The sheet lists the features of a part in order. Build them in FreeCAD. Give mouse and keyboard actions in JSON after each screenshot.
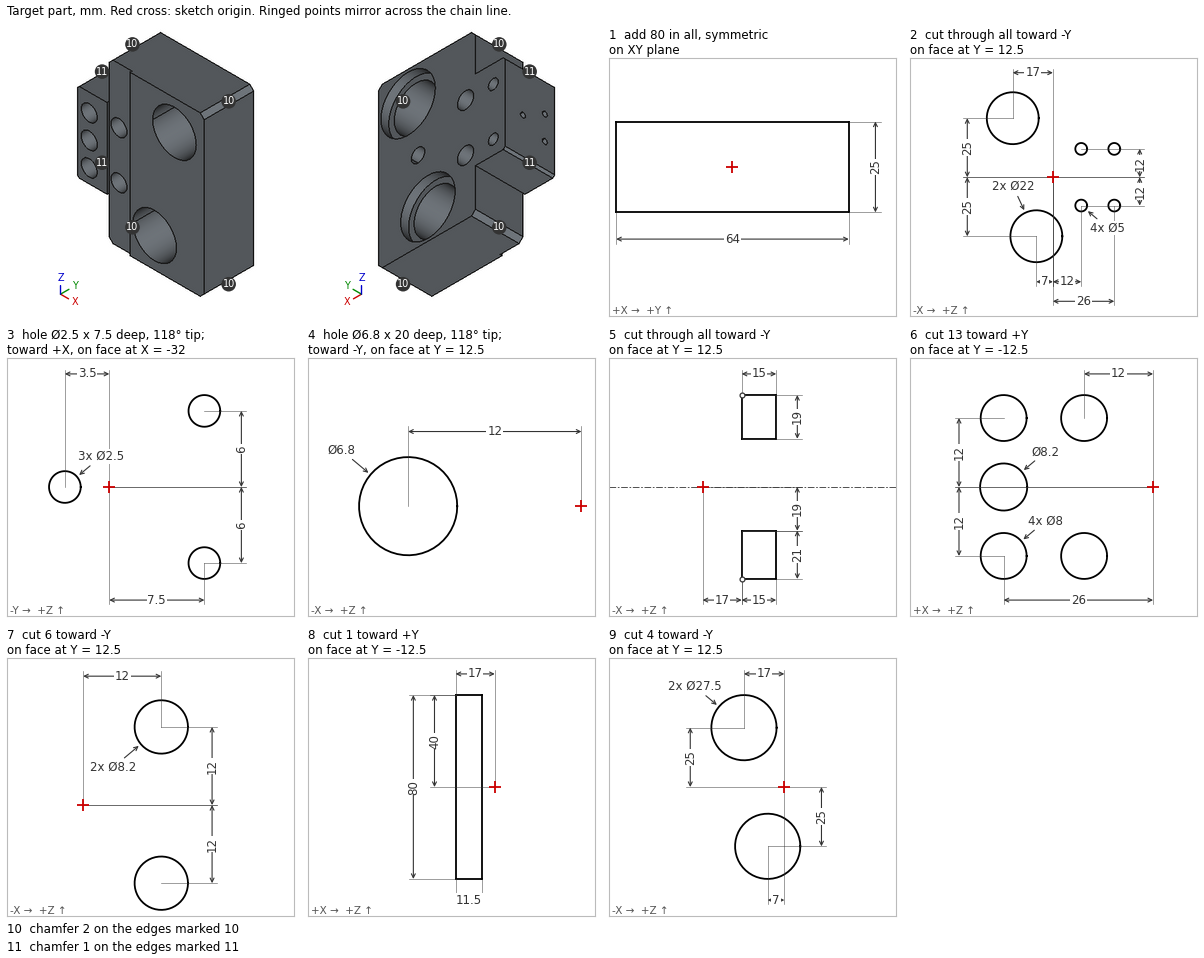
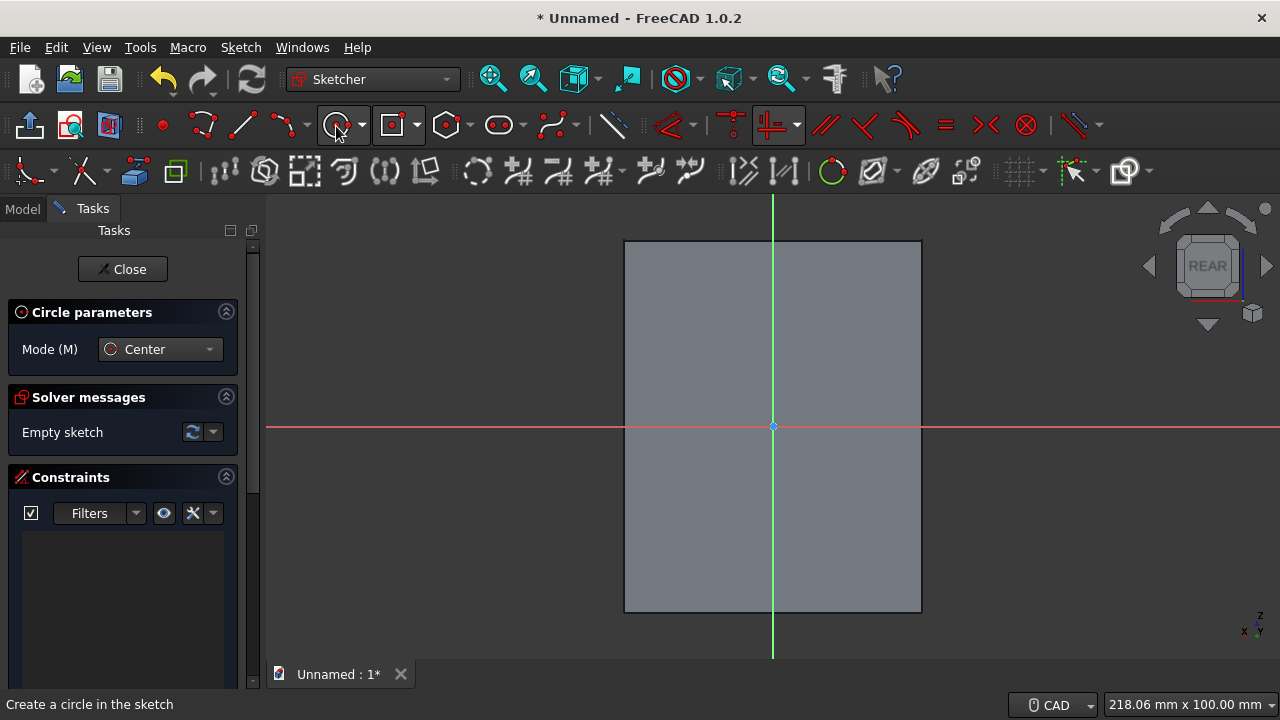
{"action": "left_click", "coordinate": [740, 543]}
{"action": "left_click", "coordinate": [704, 507]}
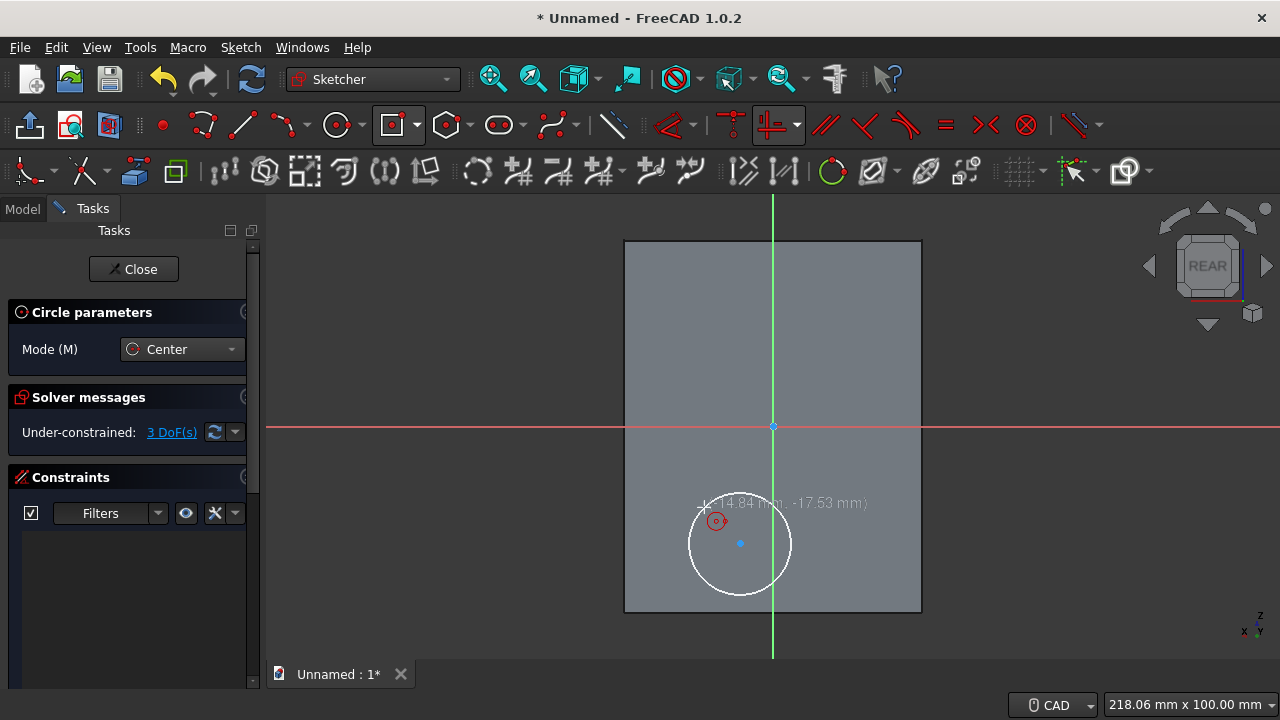
{"action": "left_click", "coordinate": [694, 310]}
{"action": "left_click", "coordinate": [730, 274]}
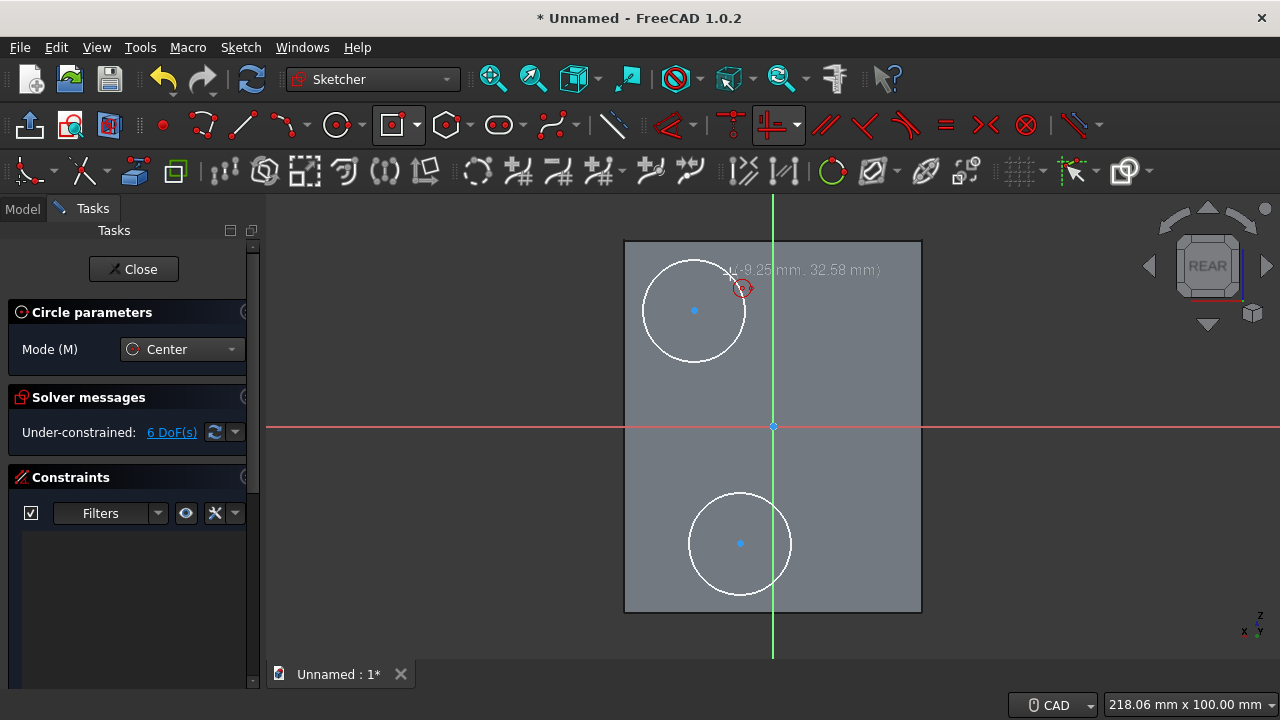
{"action": "scroll", "coordinate": [829, 482], "scroll_direction": "up", "scroll_amount": 4}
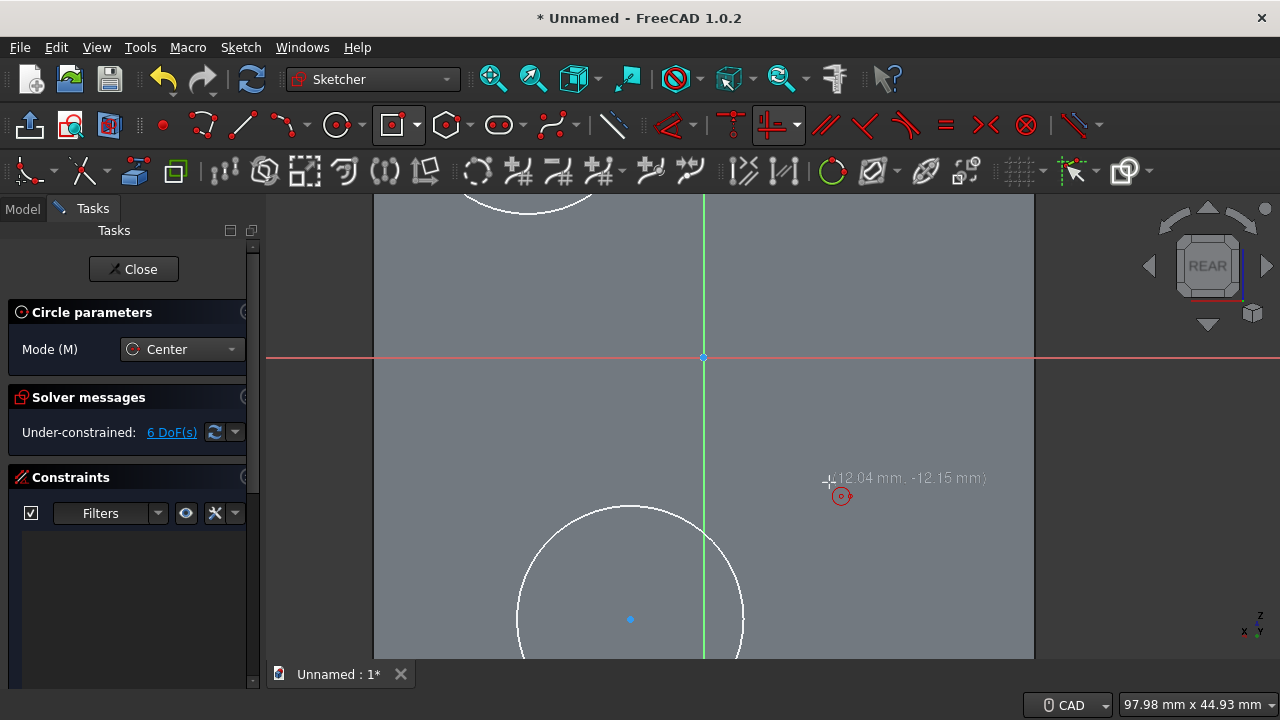
{"action": "left_click", "coordinate": [828, 482]}
{"action": "left_click", "coordinate": [846, 464]}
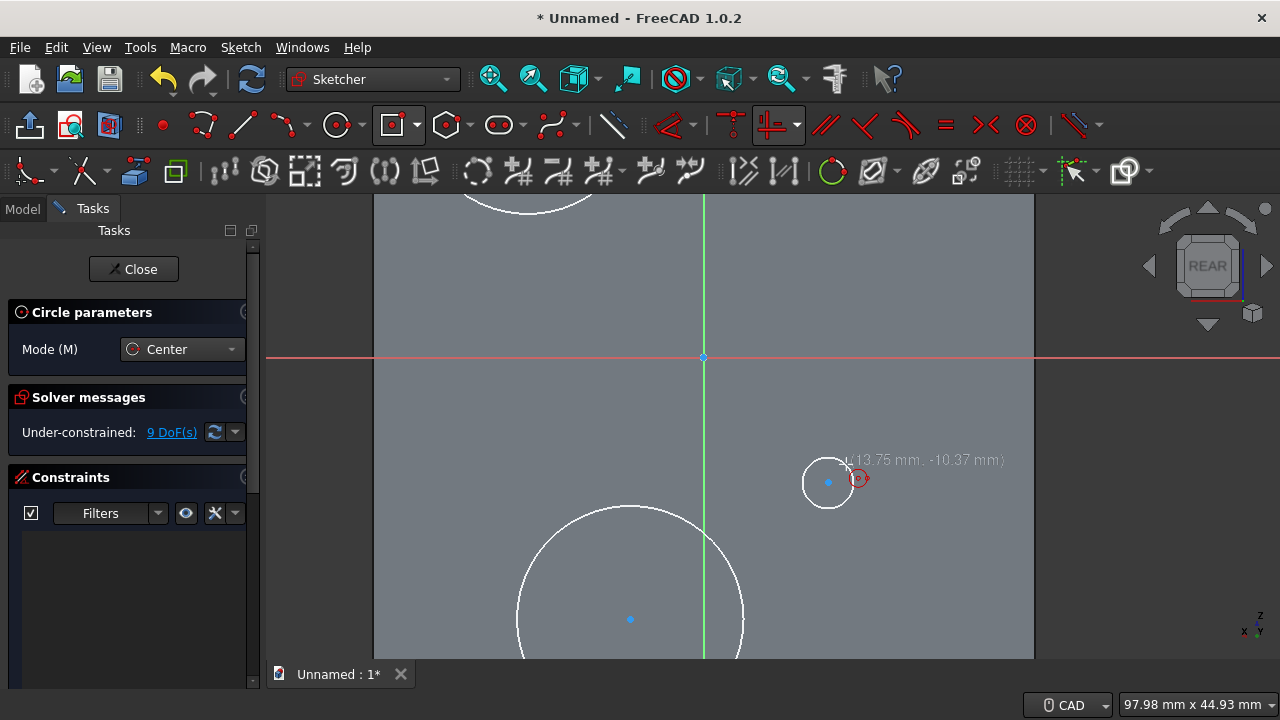
{"action": "left_click", "coordinate": [828, 234]}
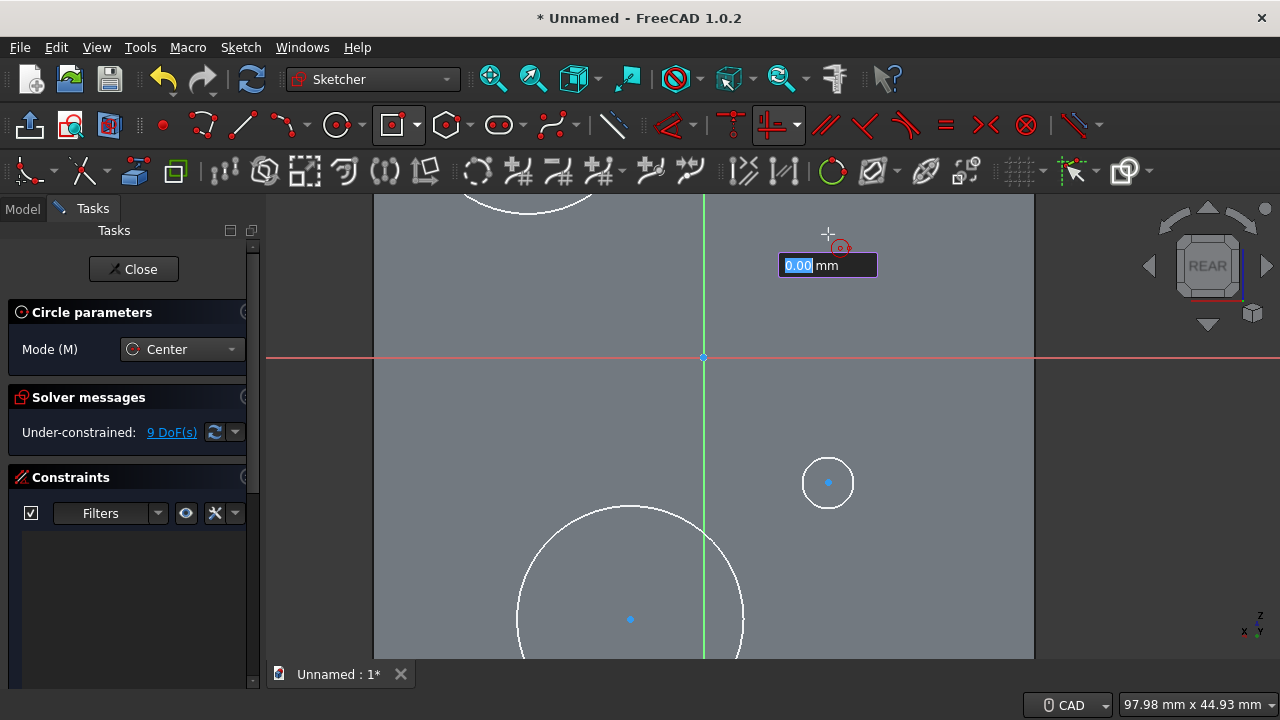
{"action": "scroll", "coordinate": [703, 467], "scroll_direction": "down", "scroll_amount": 5}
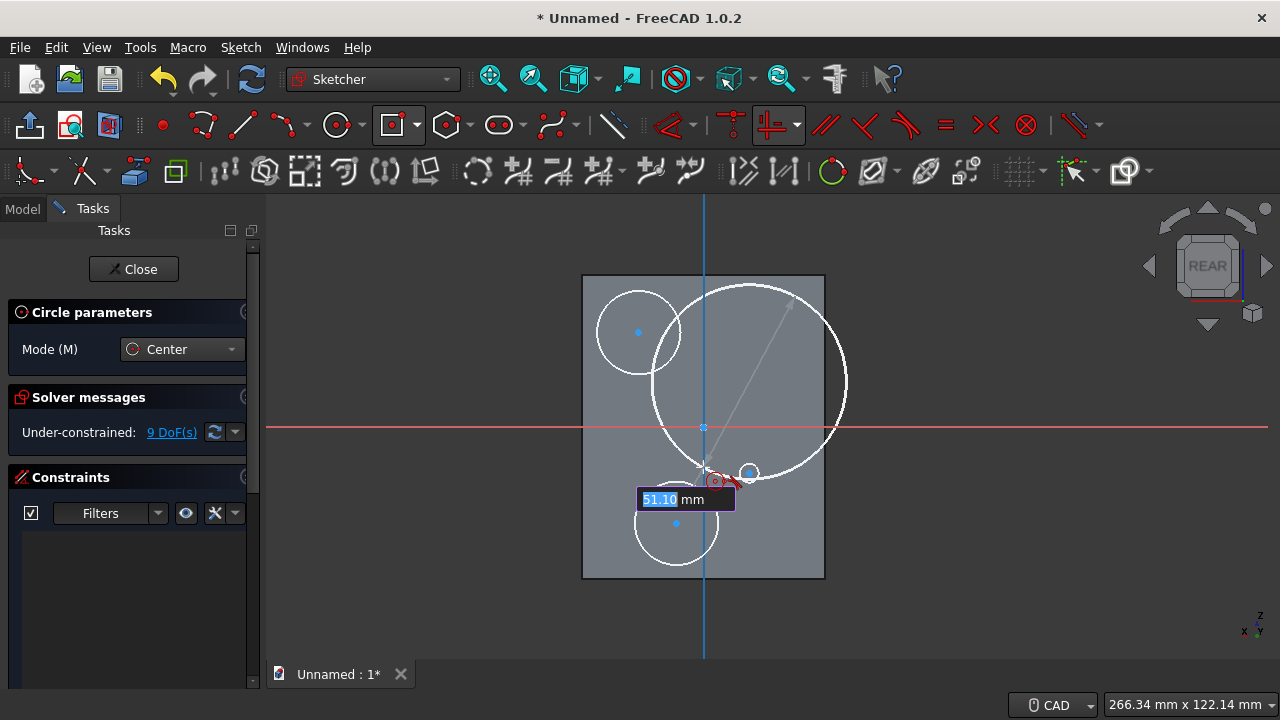
{"action": "scroll", "coordinate": [756, 375], "scroll_direction": "up", "scroll_amount": 3}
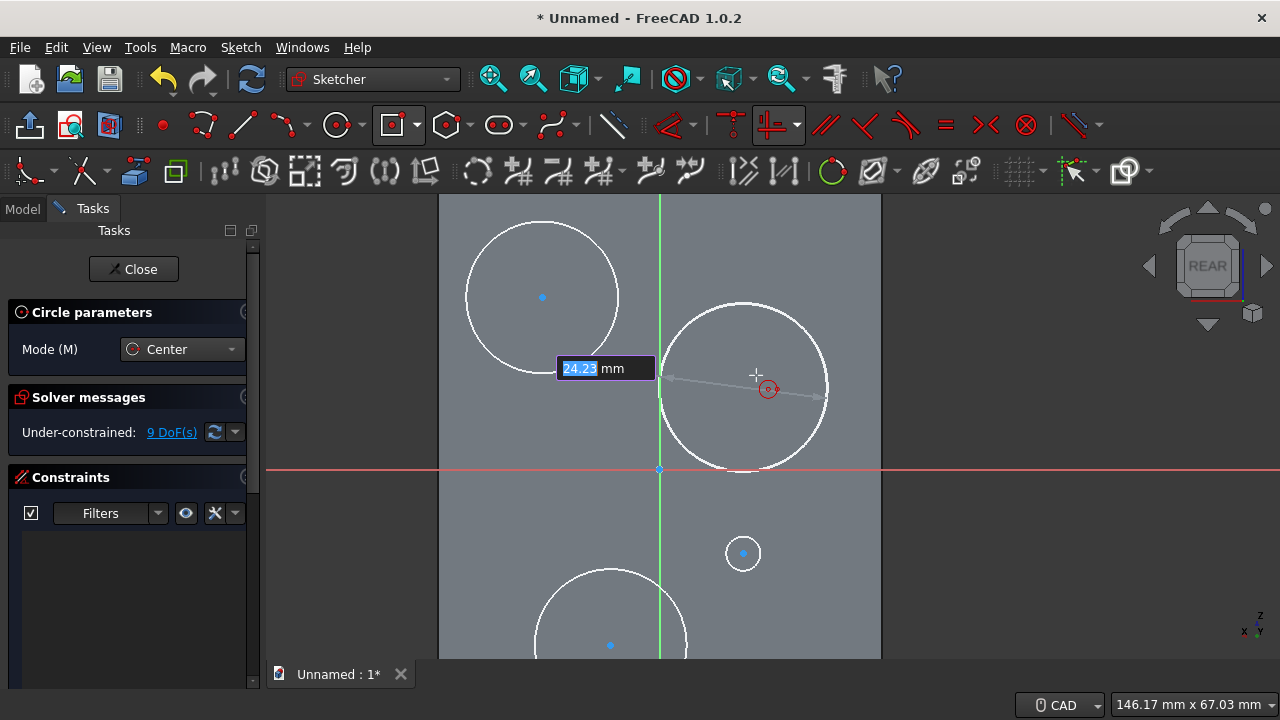
{"action": "left_click", "coordinate": [755, 374]}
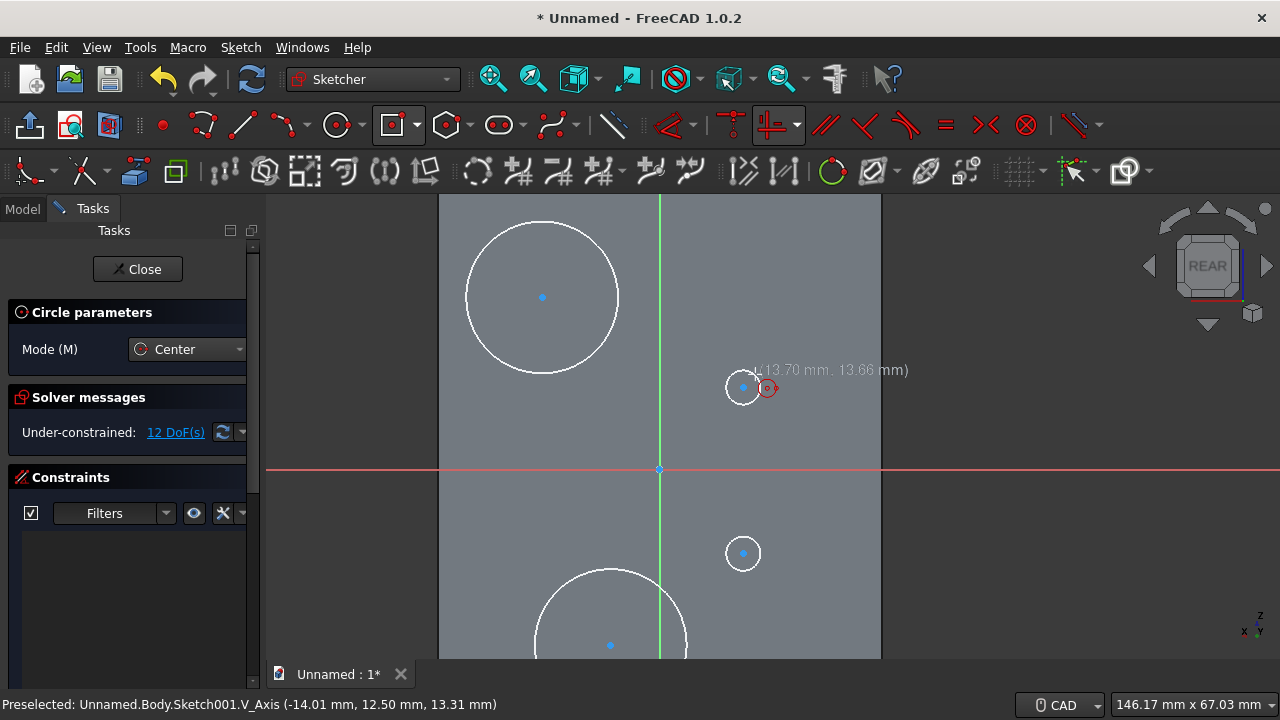
{"action": "scroll", "coordinate": [840, 553], "scroll_direction": "up", "scroll_amount": 2}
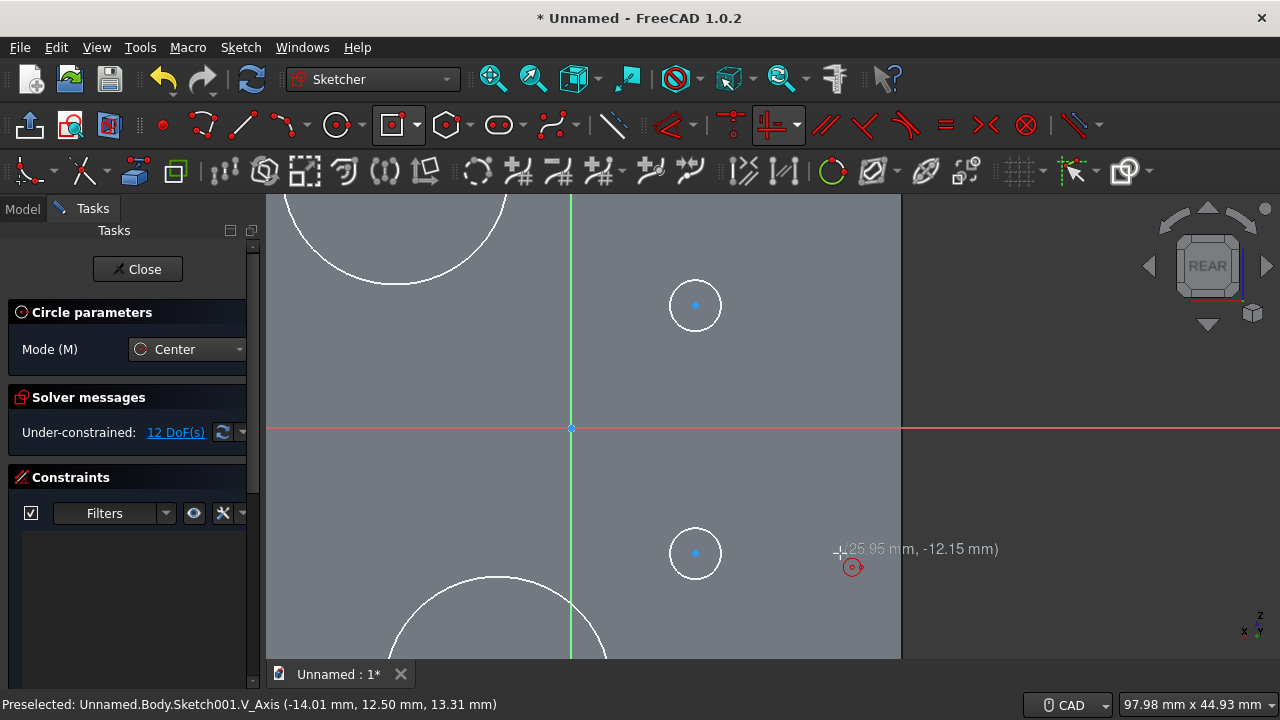
{"action": "left_click", "coordinate": [840, 553]}
{"action": "left_click", "coordinate": [859, 534]}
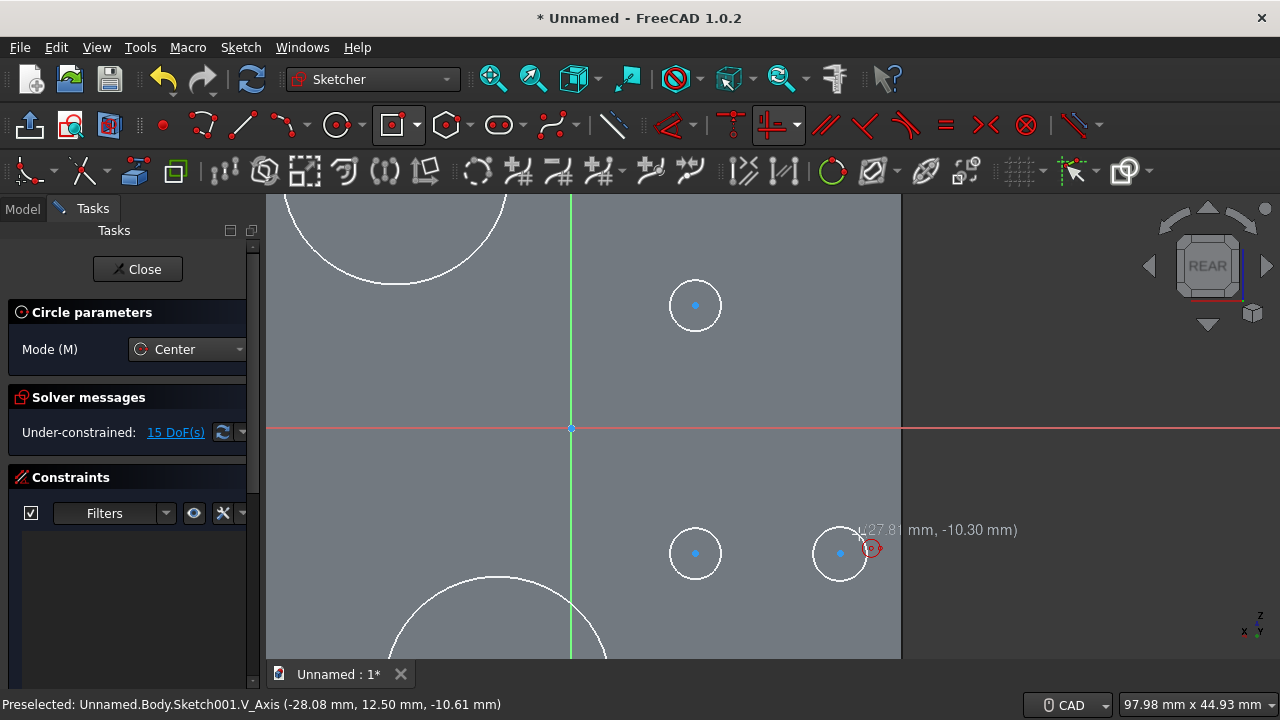
{"action": "left_click", "coordinate": [840, 304]}
{"action": "left_click", "coordinate": [859, 286]}
{"action": "key", "text": "Escape"}